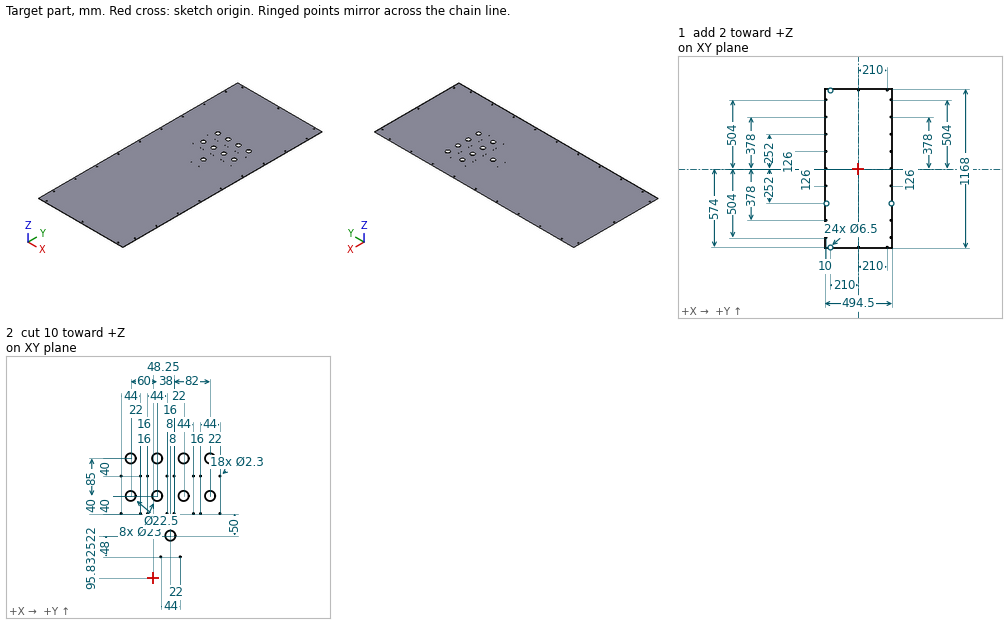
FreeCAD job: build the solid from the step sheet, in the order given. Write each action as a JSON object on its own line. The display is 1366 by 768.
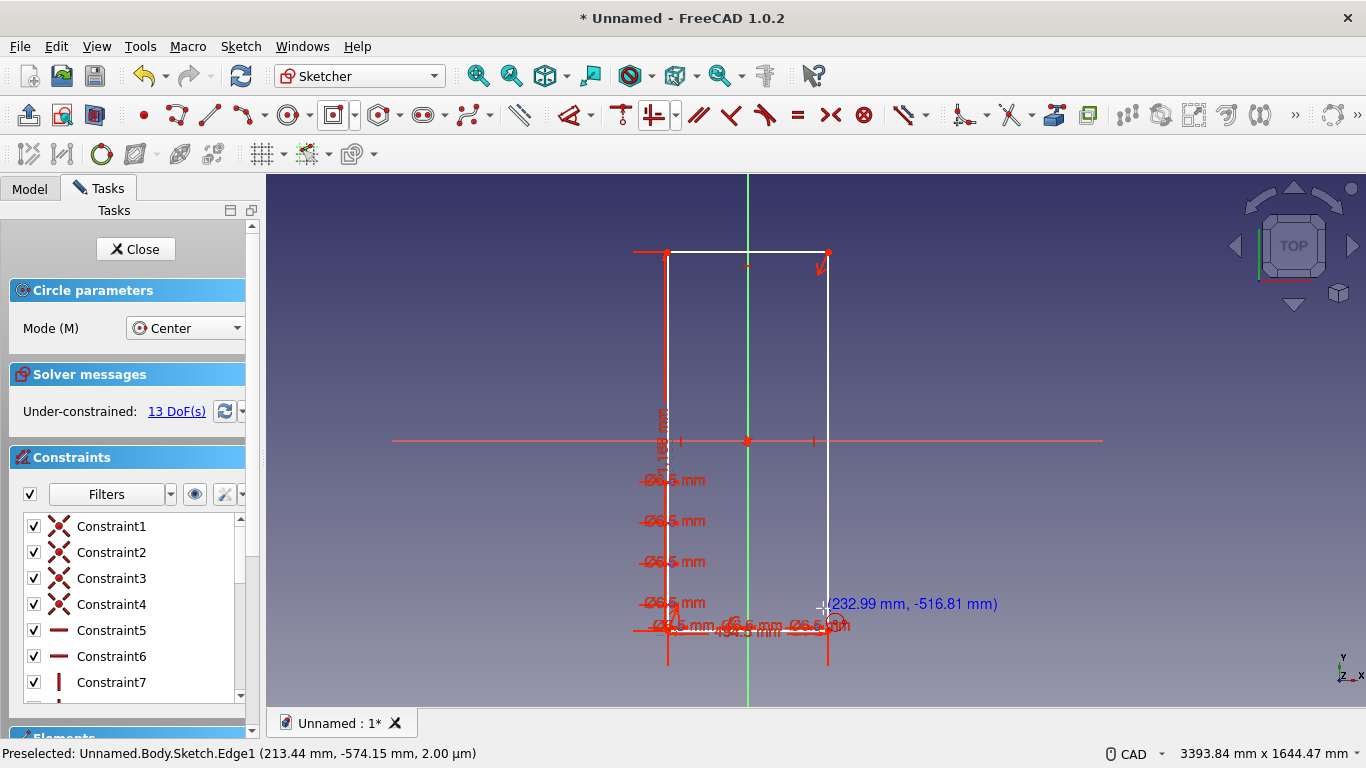
{"action": "scroll", "coordinate": [825, 605], "scroll_direction": "up", "scroll_amount": 8}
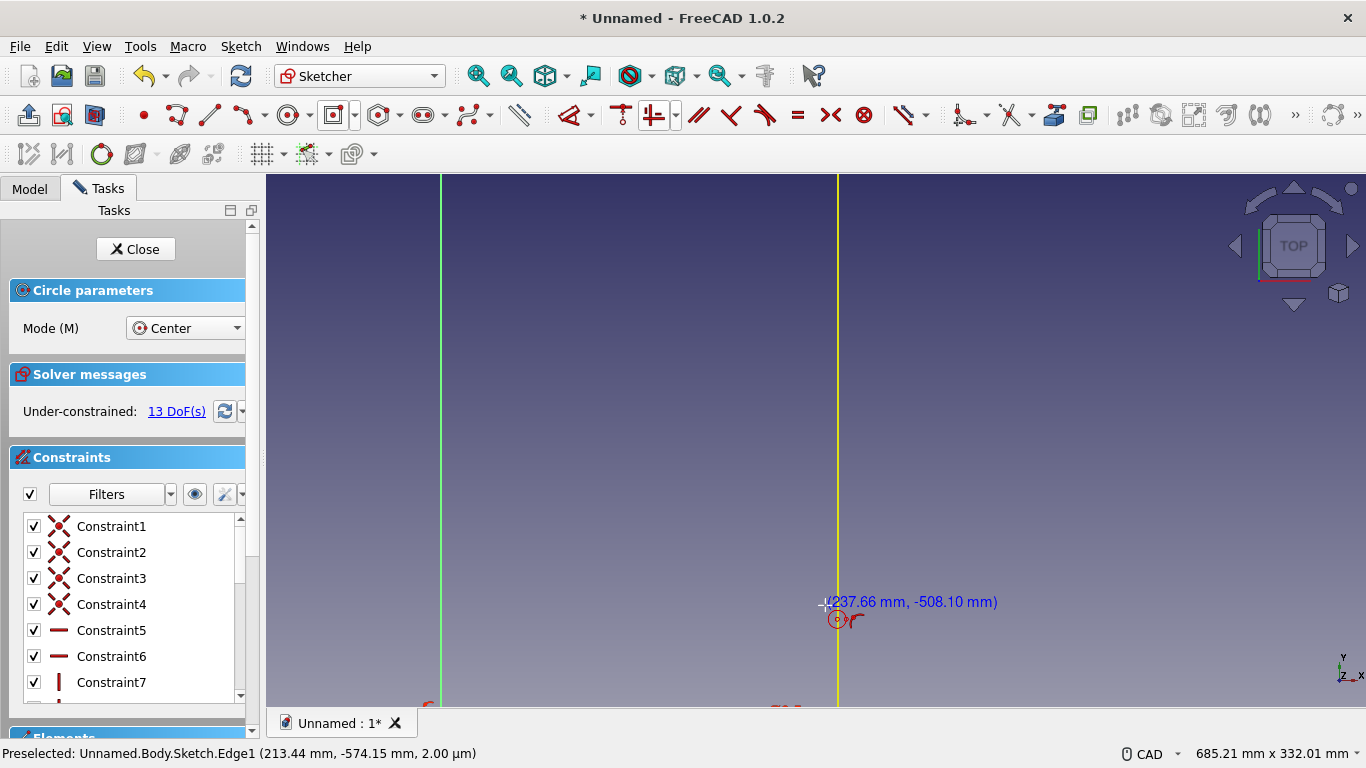
{"action": "left_click", "coordinate": [822, 600]}
{"action": "mouse_move", "coordinate": [819, 596]}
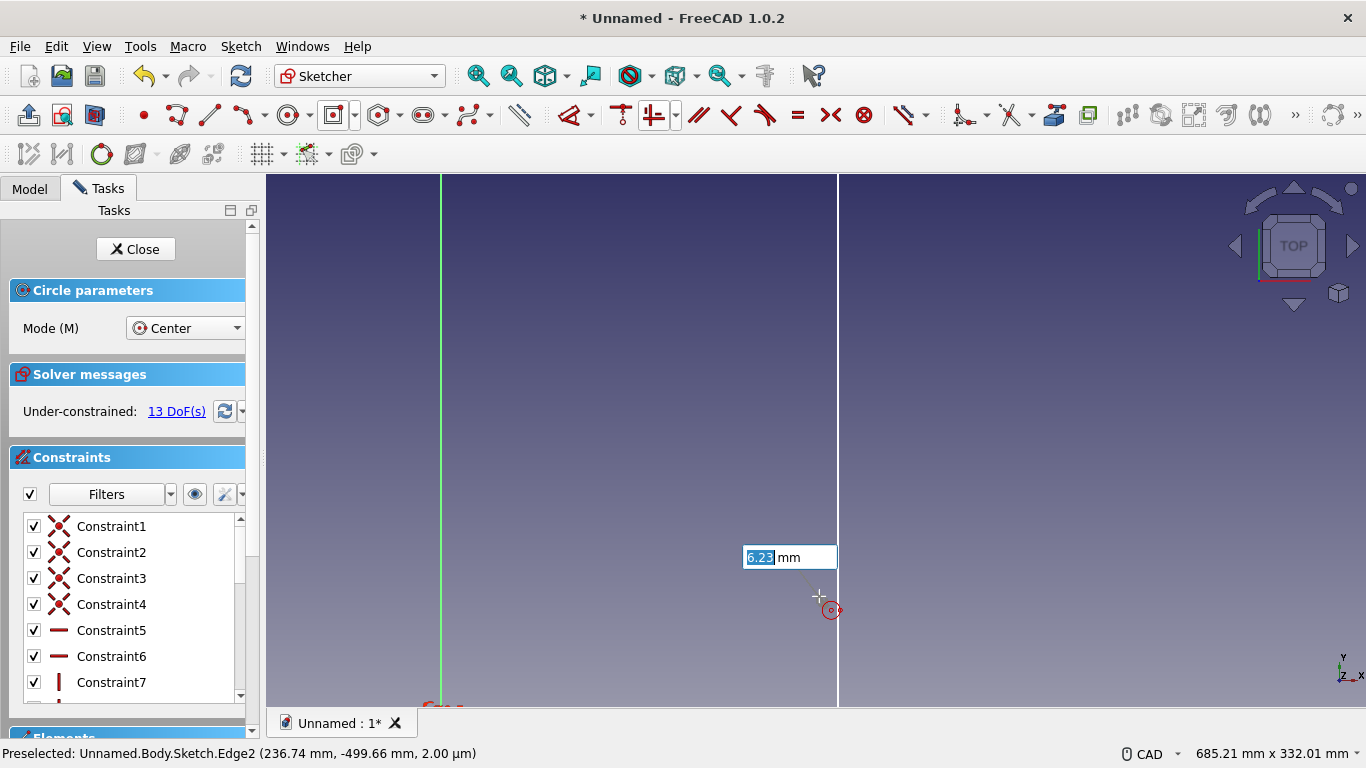
{"action": "type", "text": "6.5"}
{"action": "key", "text": "Return"}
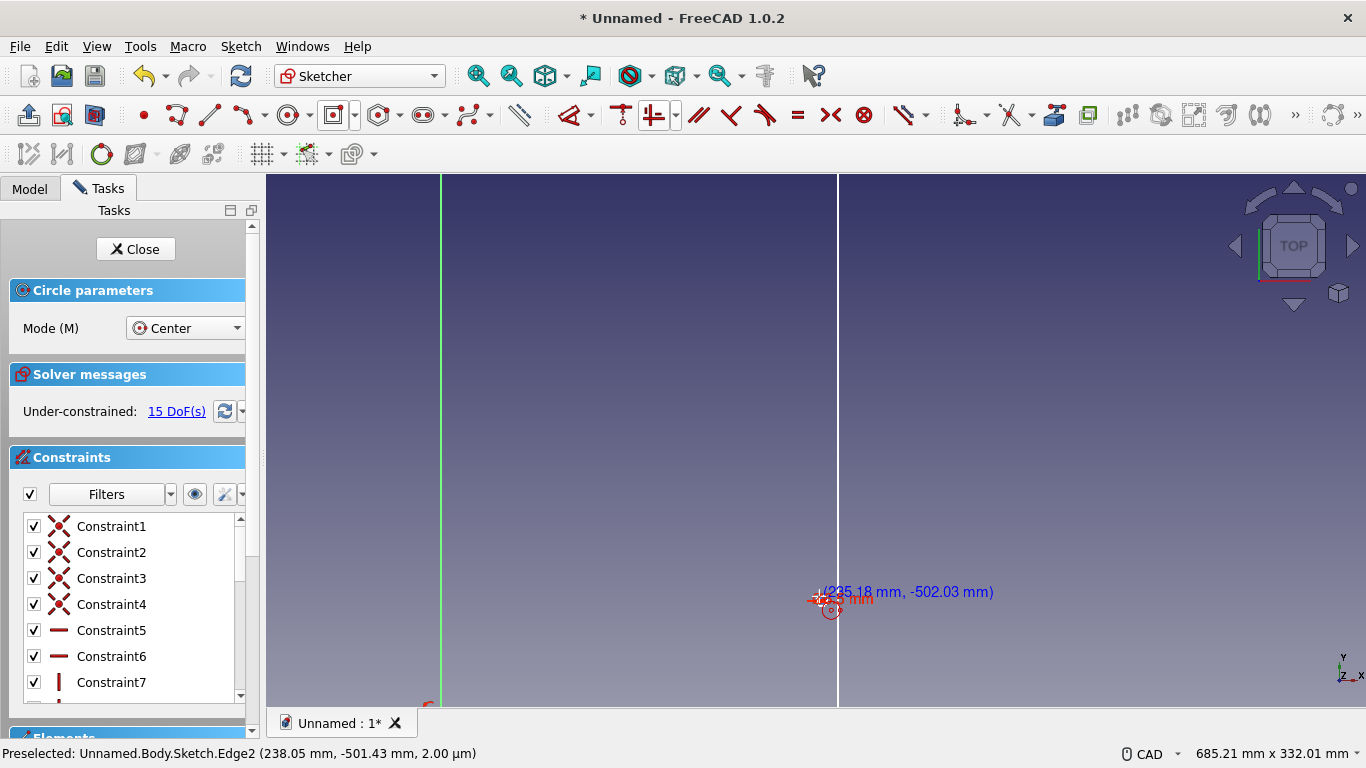
{"action": "scroll", "coordinate": [822, 398], "scroll_direction": "up", "scroll_amount": 8}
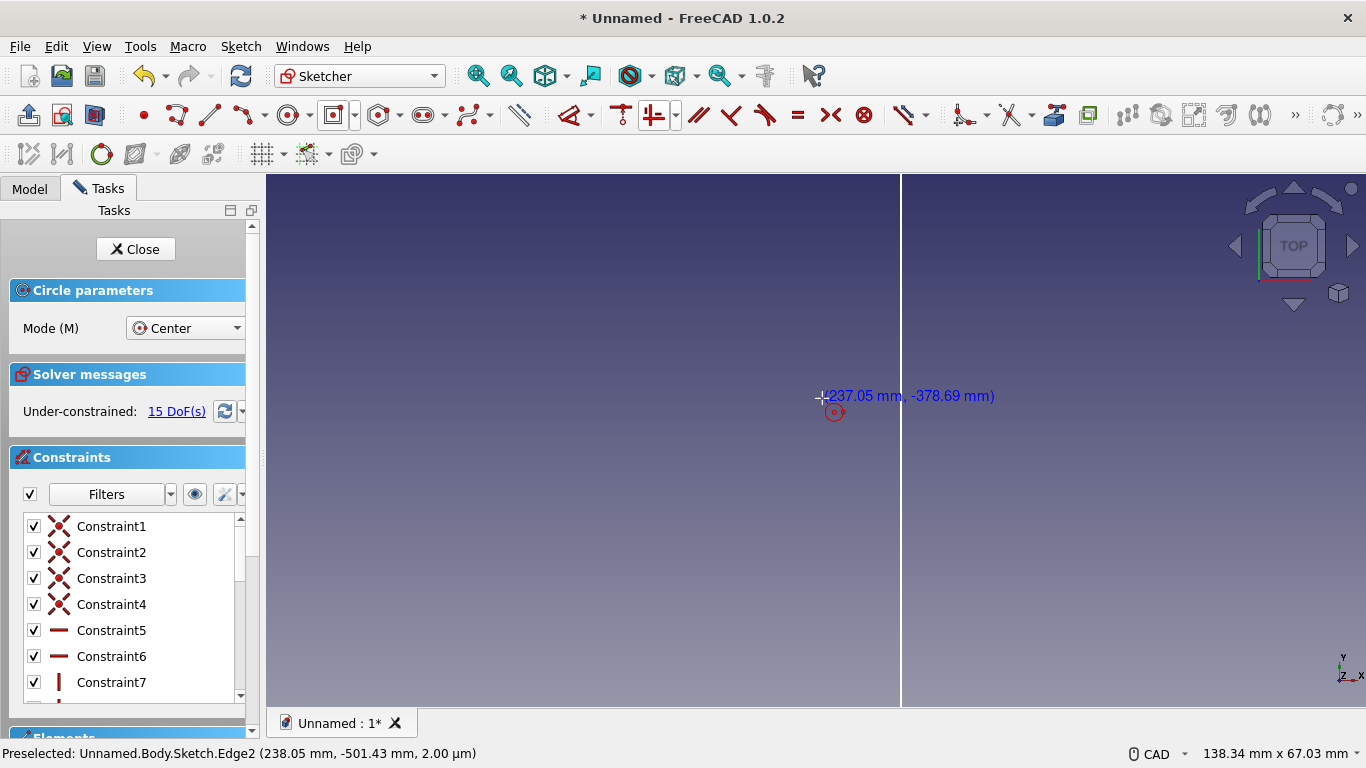
{"action": "scroll", "coordinate": [825, 570], "scroll_direction": "down", "scroll_amount": 16}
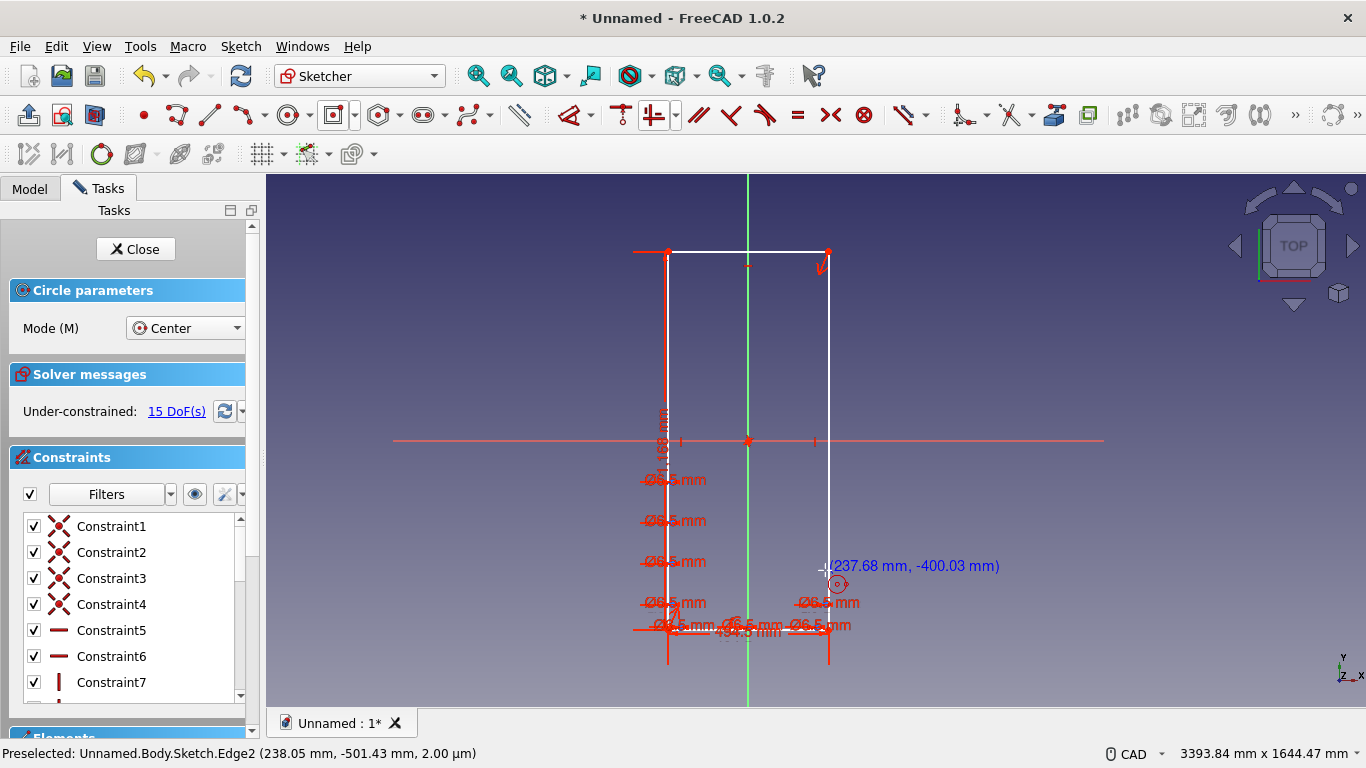
{"action": "scroll", "coordinate": [825, 564], "scroll_direction": "up", "scroll_amount": 8}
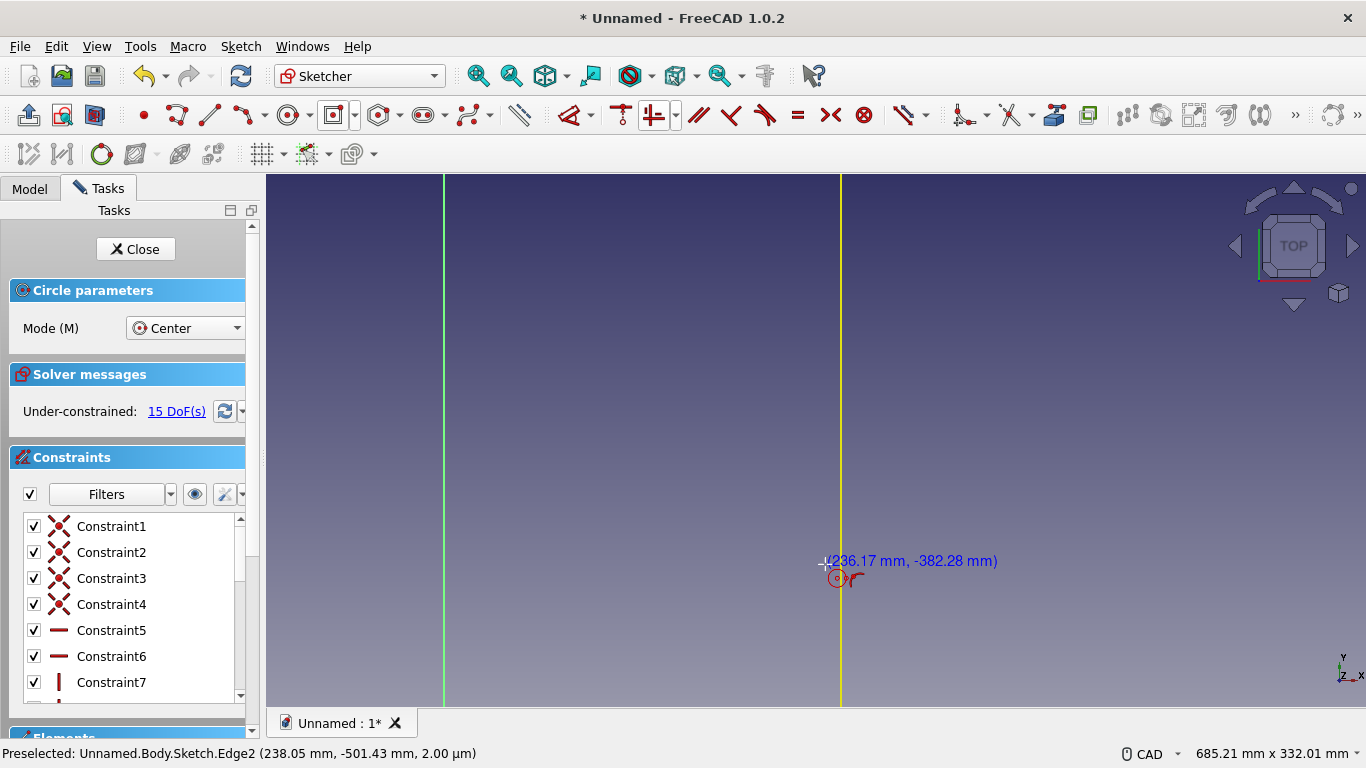
{"action": "left_click", "coordinate": [825, 559]}
{"action": "mouse_move", "coordinate": [821, 556]}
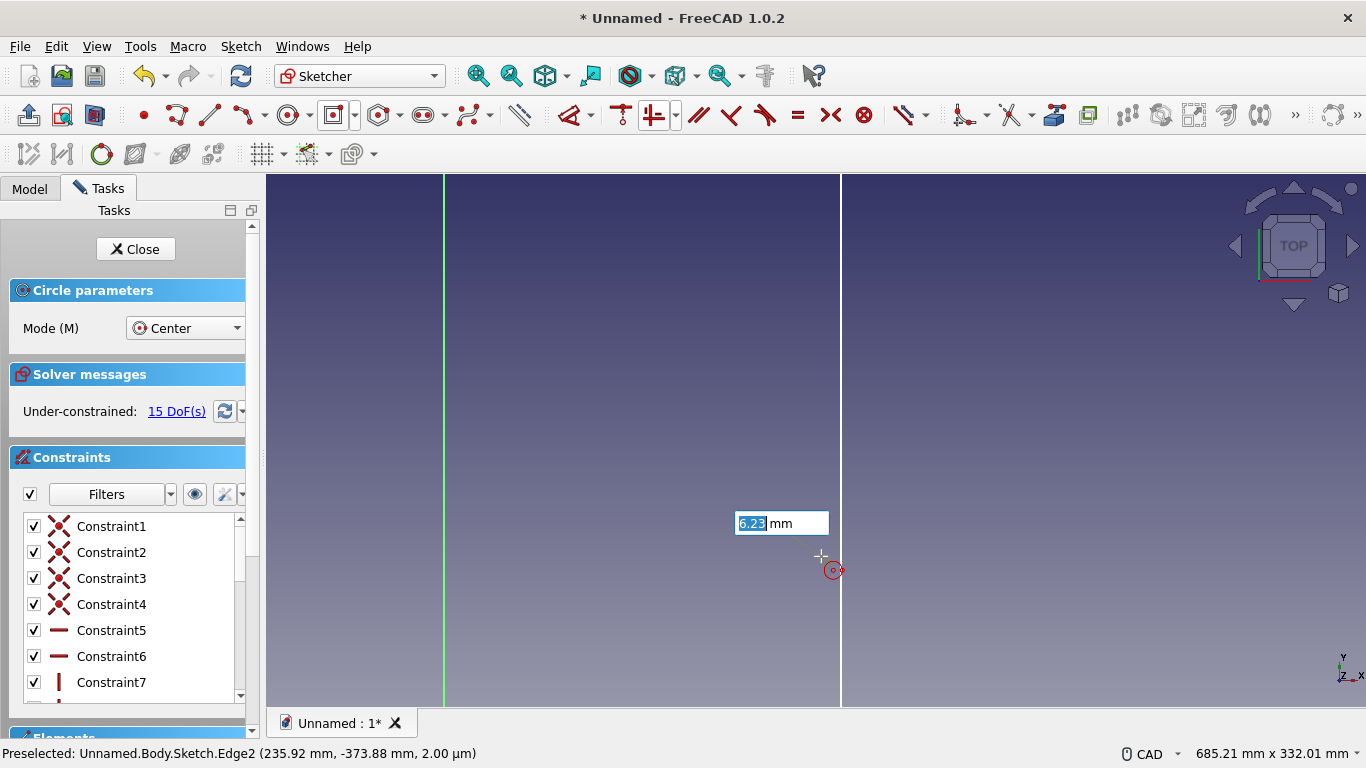
{"action": "type", "text": "6.5"}
{"action": "key", "text": "Return"}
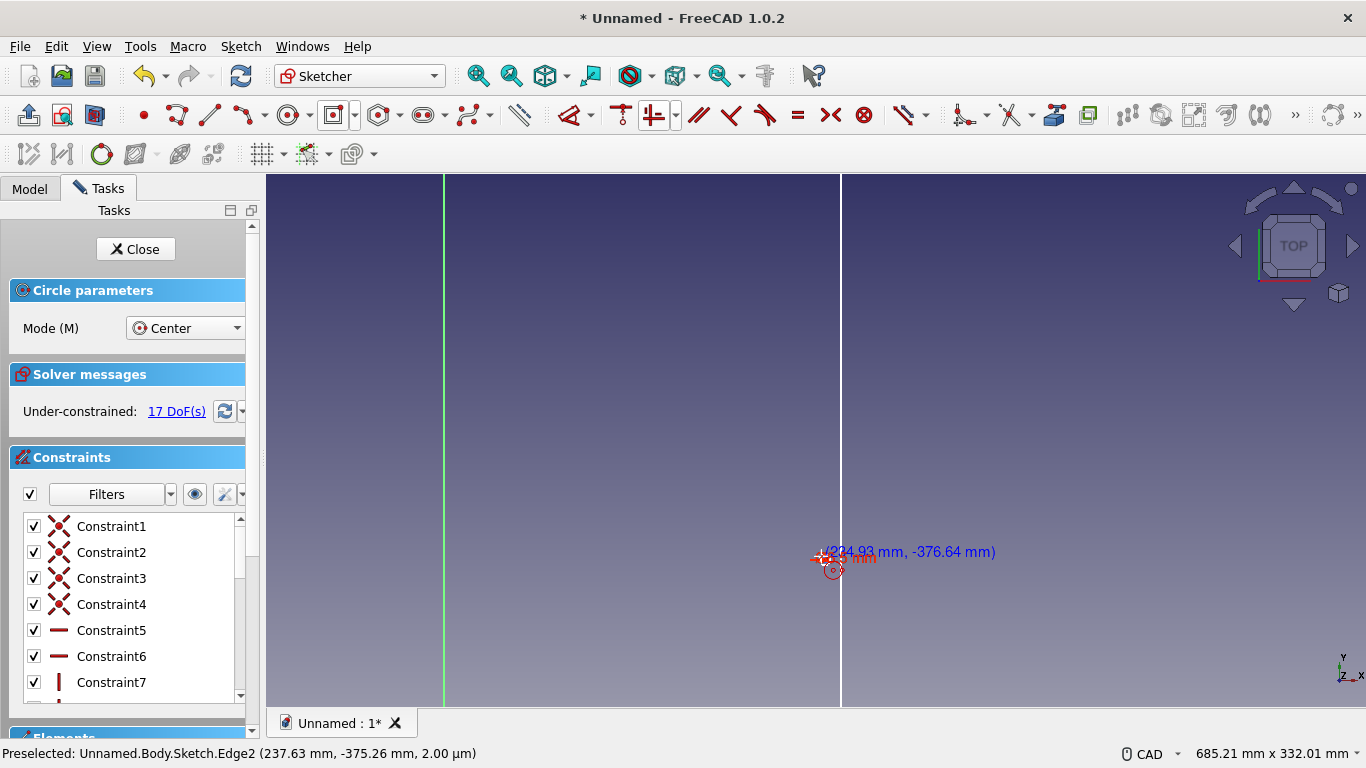
{"action": "scroll", "coordinate": [825, 357], "scroll_direction": "up", "scroll_amount": 8}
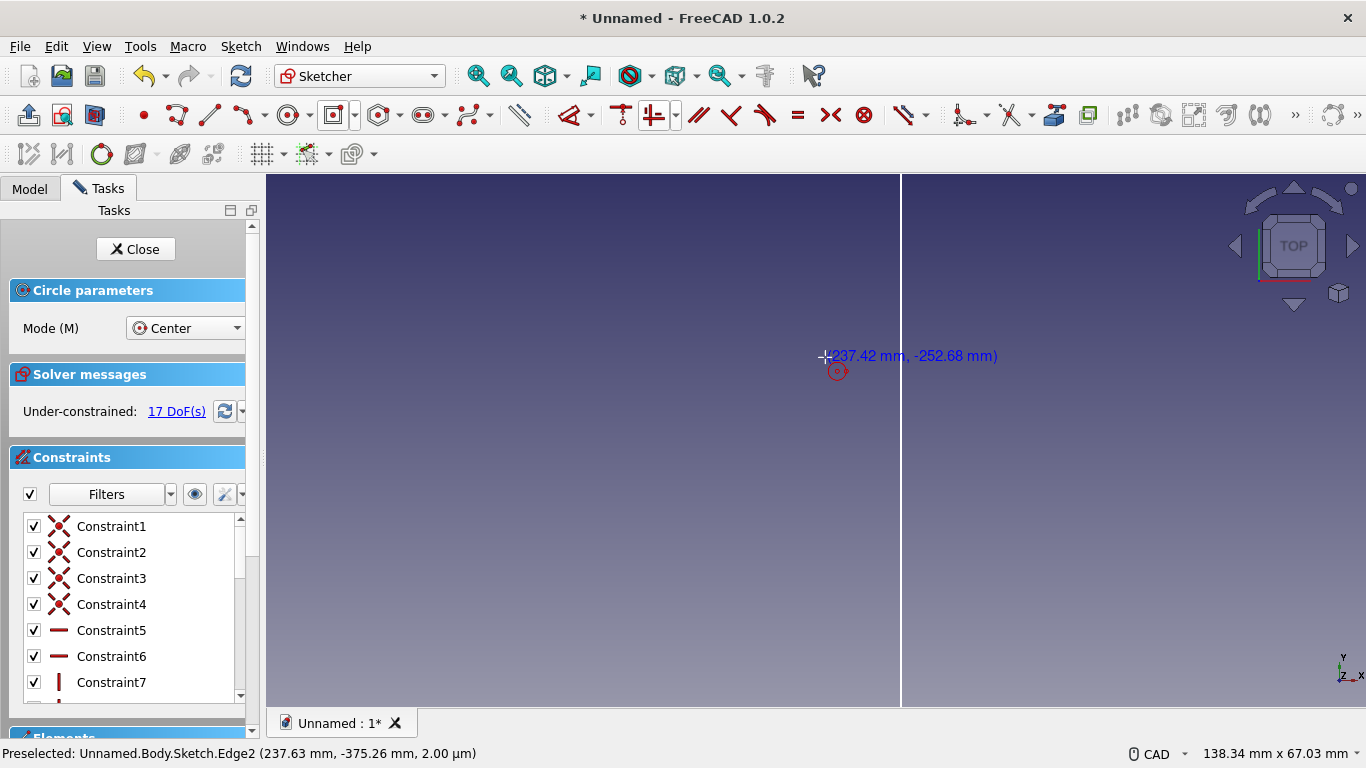
{"action": "scroll", "coordinate": [825, 529], "scroll_direction": "down", "scroll_amount": 16}